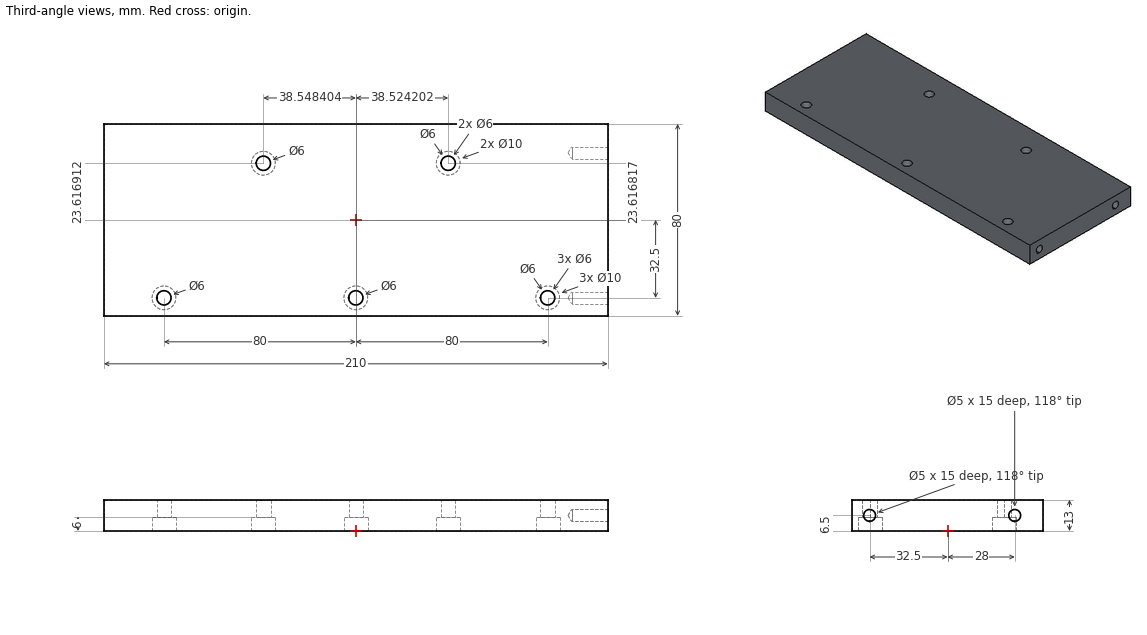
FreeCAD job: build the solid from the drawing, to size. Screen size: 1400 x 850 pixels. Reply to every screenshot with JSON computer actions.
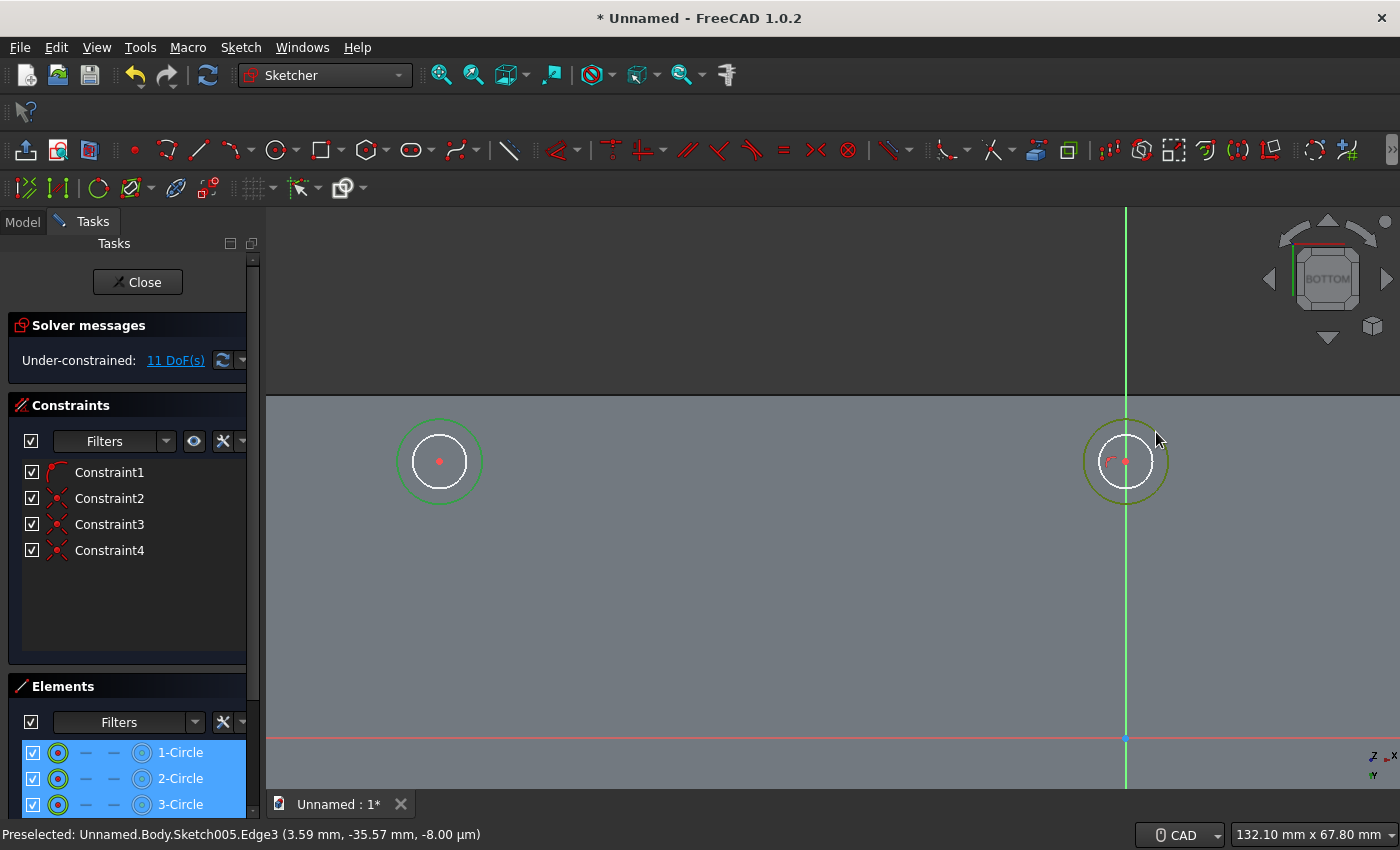
{"action": "key", "text": "e"}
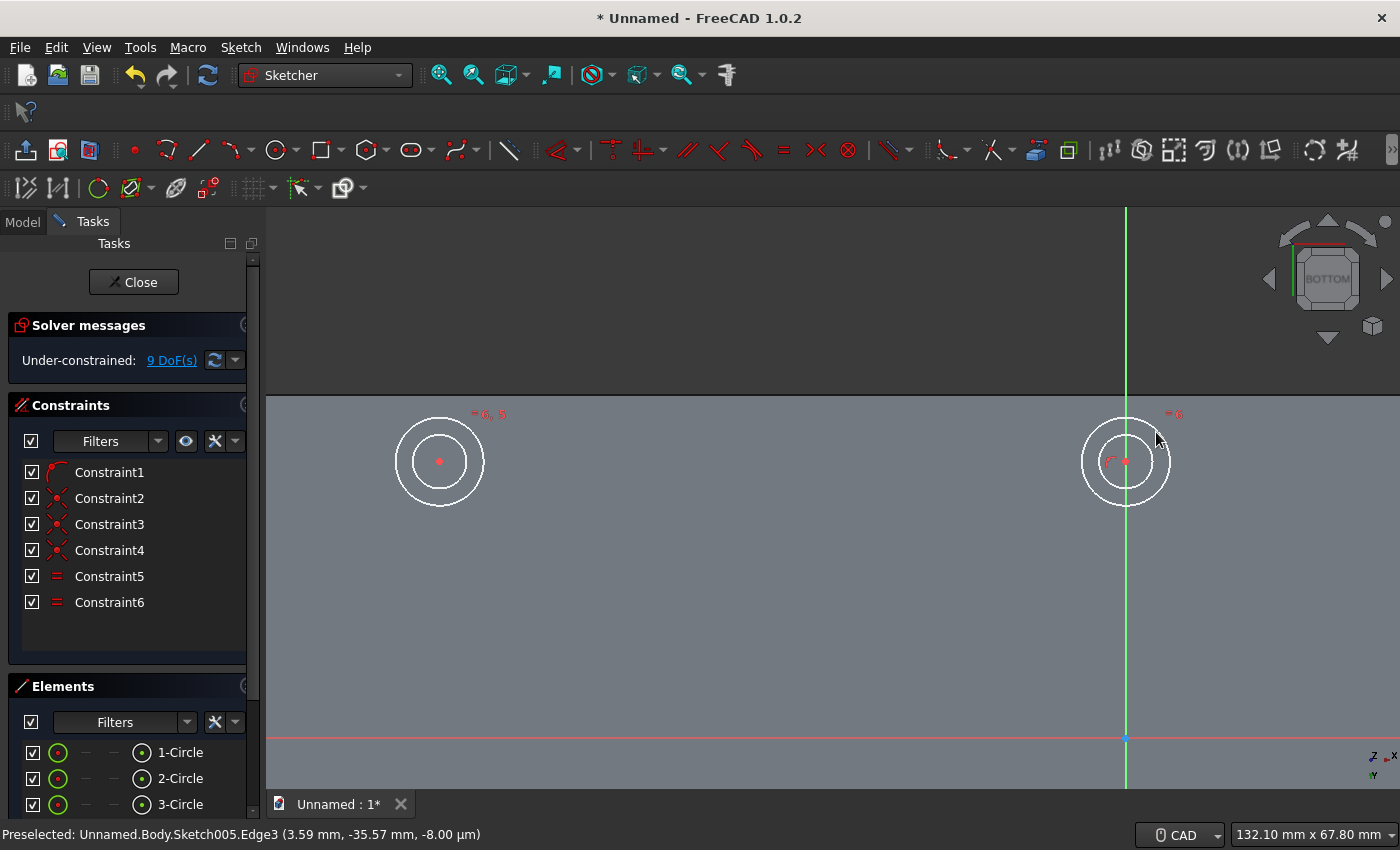
{"action": "scroll", "coordinate": [470, 433], "scroll_direction": "down", "scroll_amount": 4}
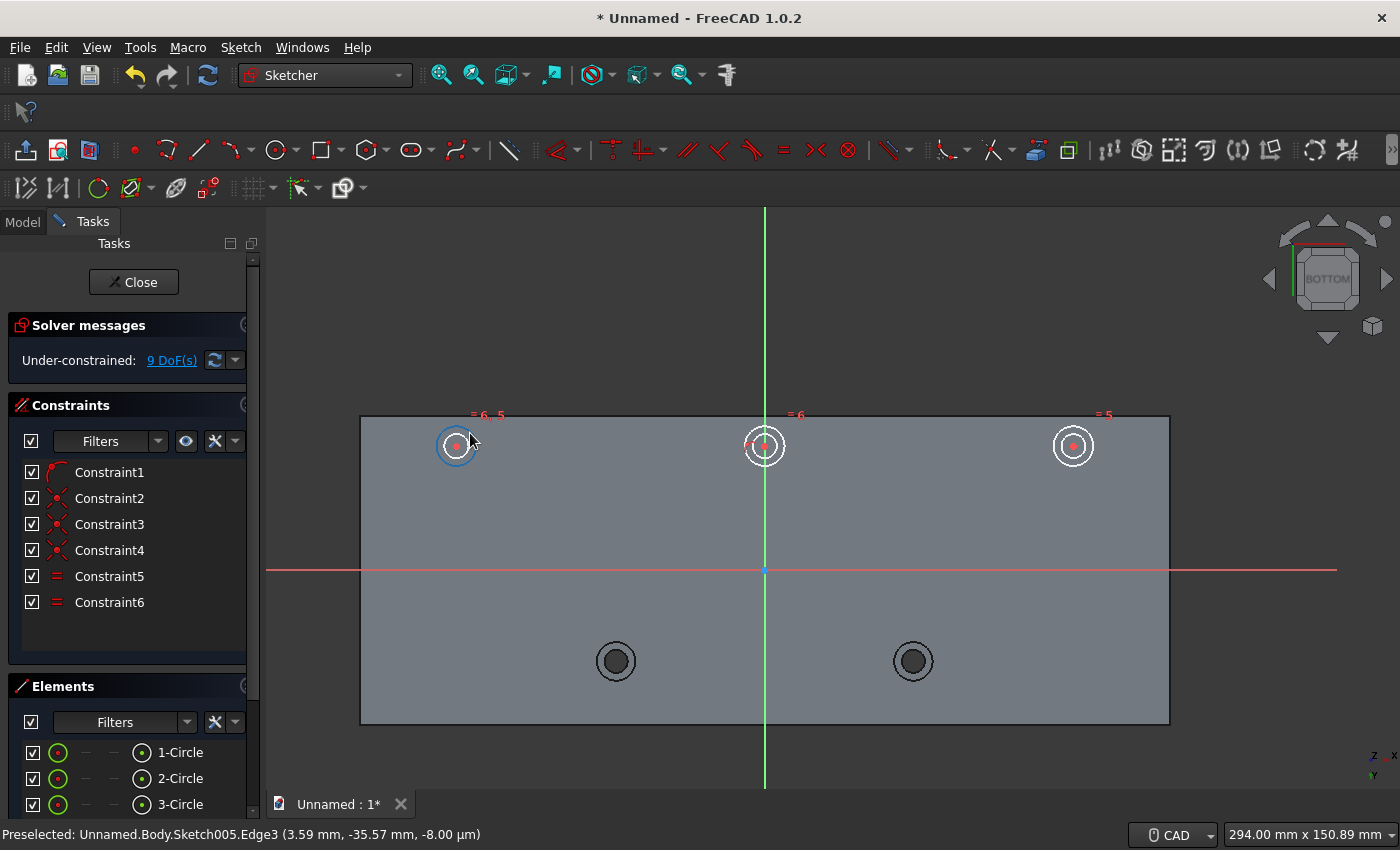
{"action": "scroll", "coordinate": [1082, 438], "scroll_direction": "up", "scroll_amount": 3}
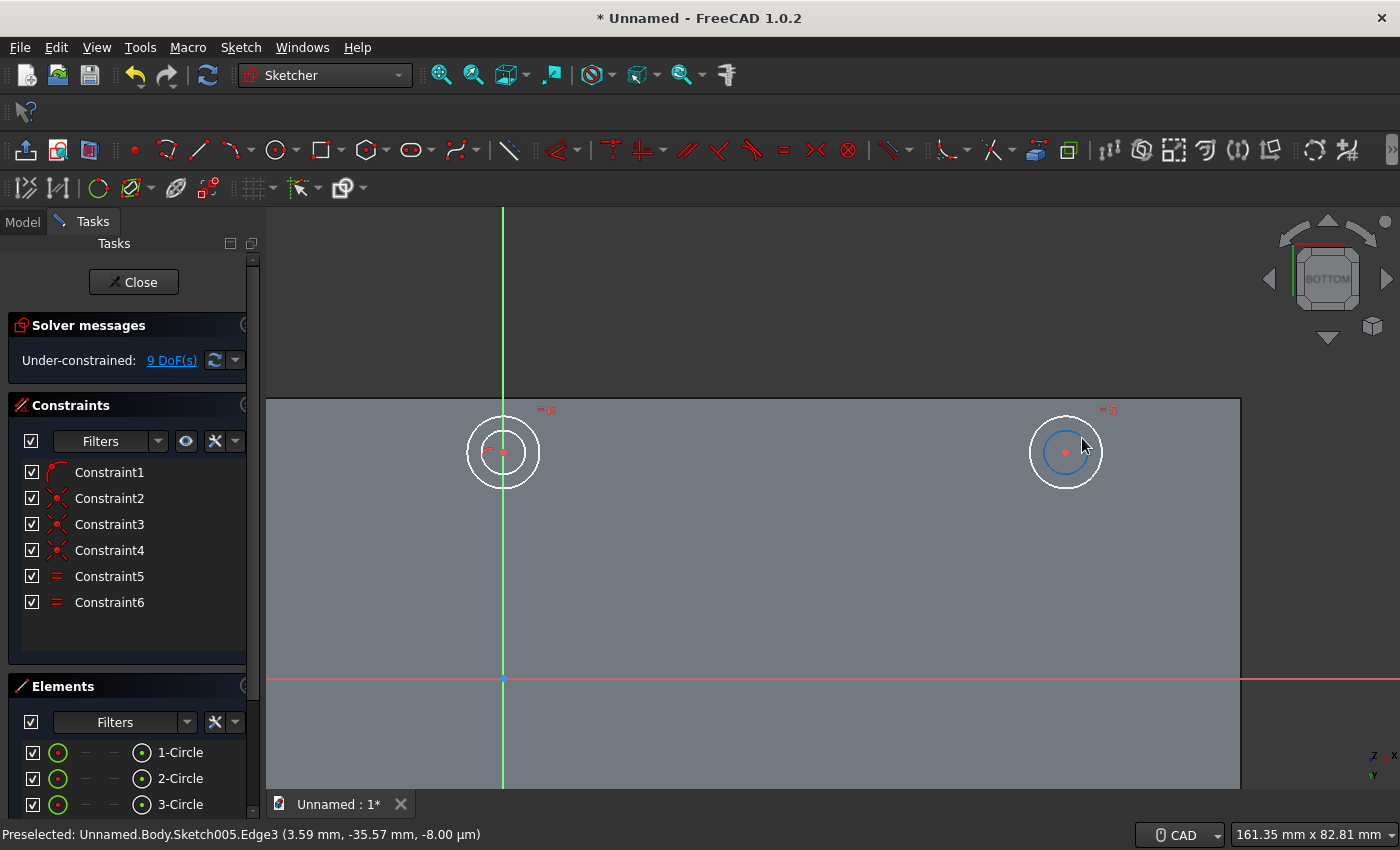
{"action": "left_click", "coordinate": [1081, 437]}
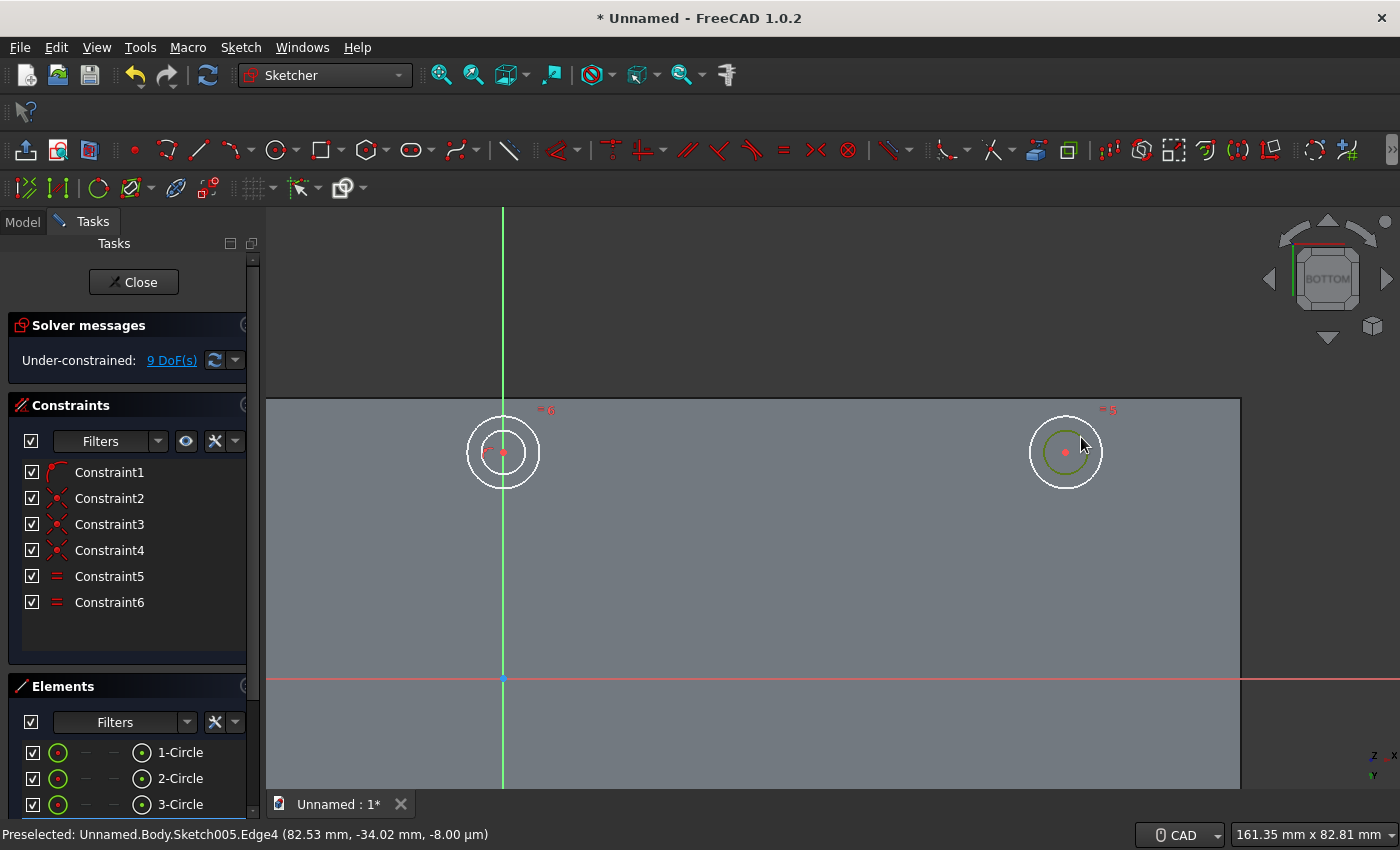
{"action": "scroll", "coordinate": [1082, 438], "scroll_direction": "down", "scroll_amount": 3}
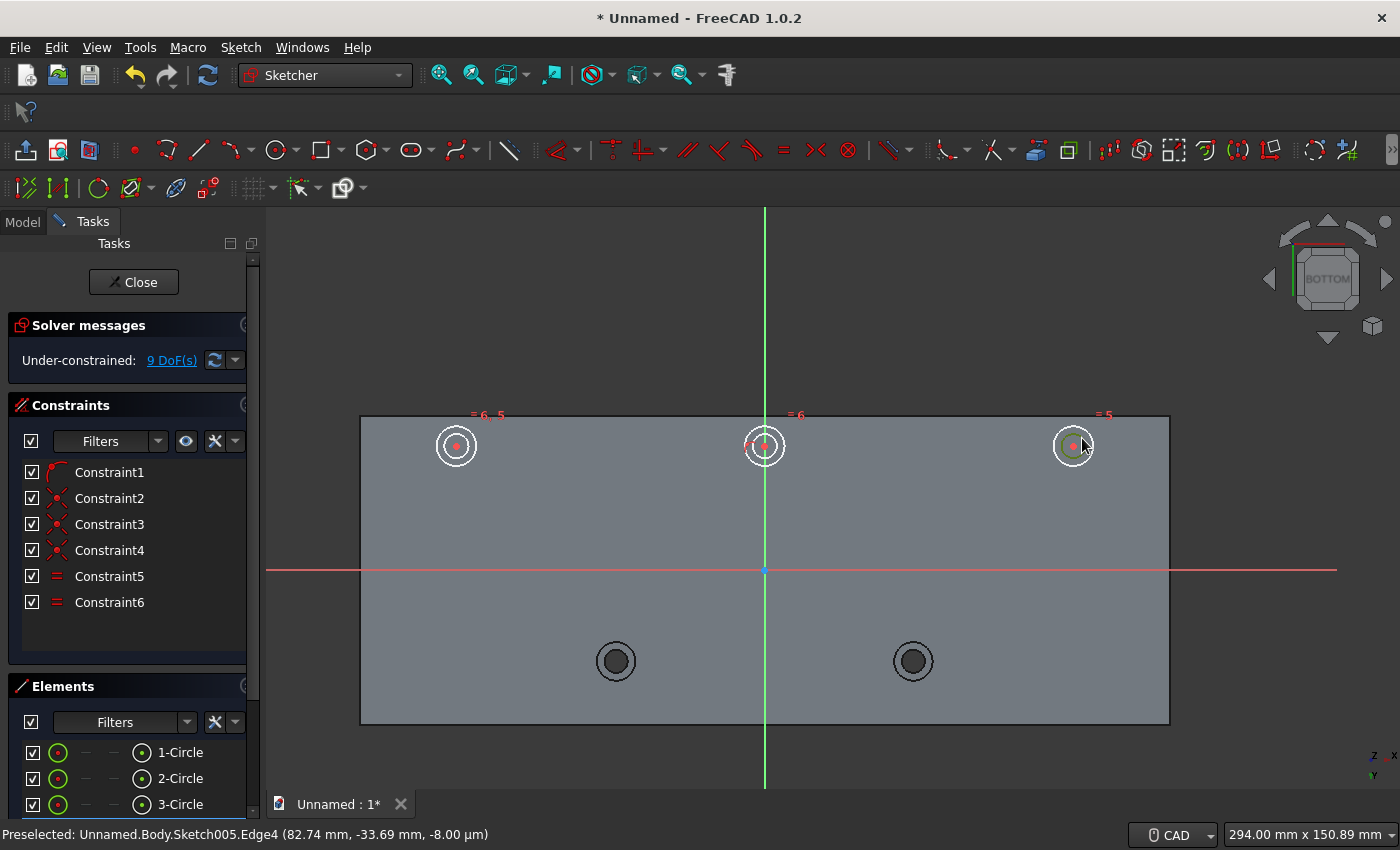
{"action": "scroll", "coordinate": [465, 438], "scroll_direction": "up", "scroll_amount": 3}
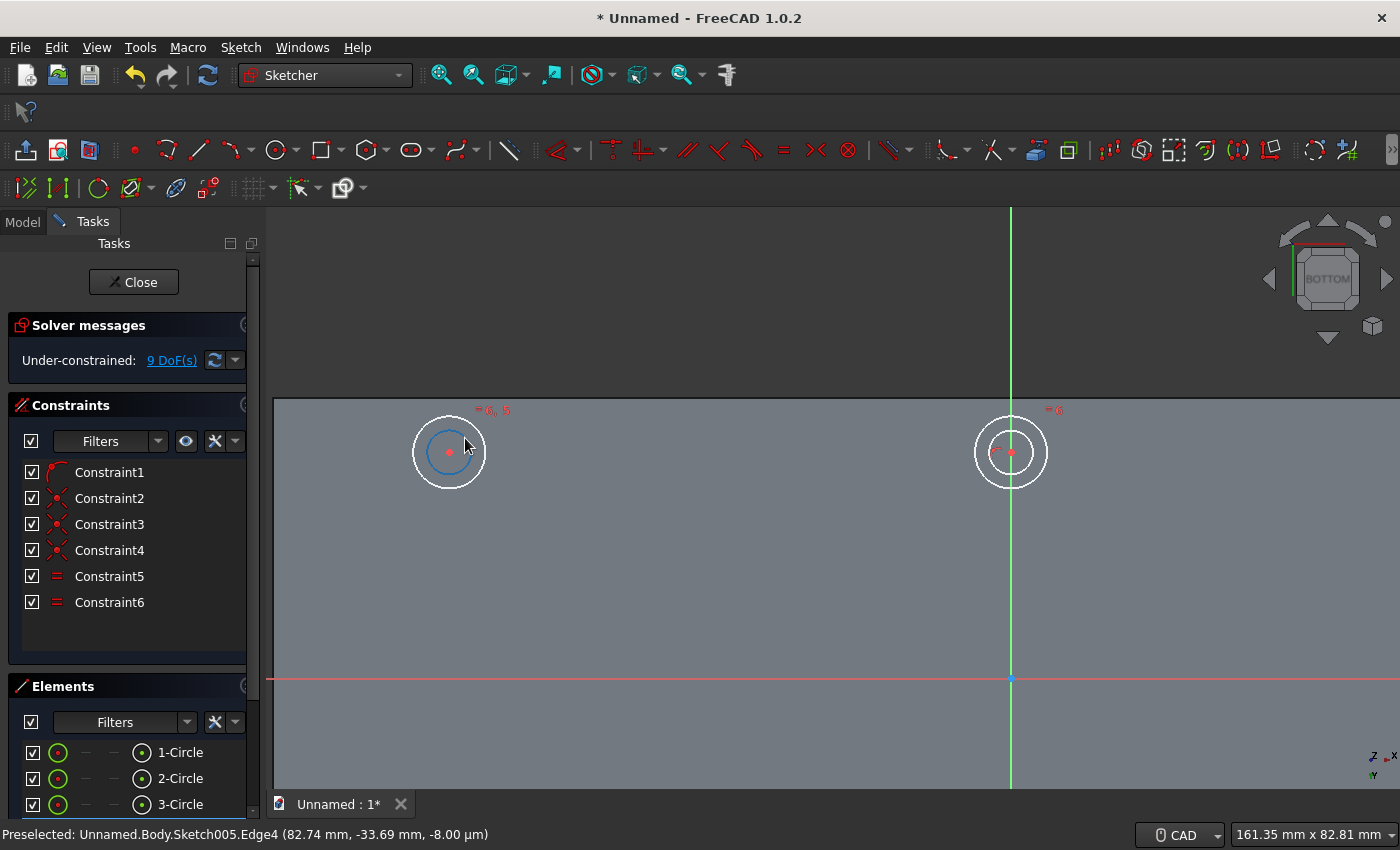
{"action": "left_click", "coordinate": [465, 437]}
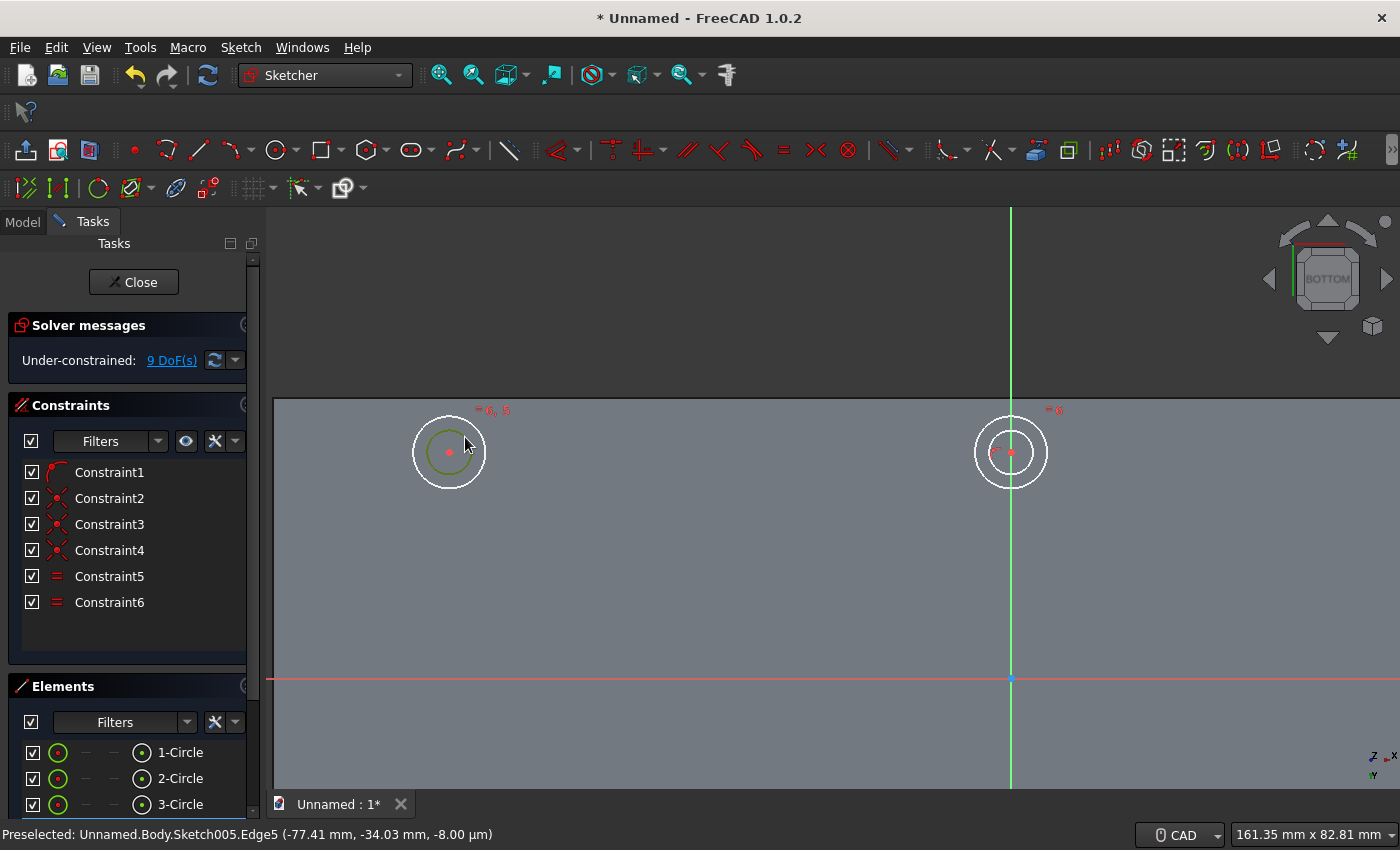
{"action": "left_click", "coordinate": [1027, 437]}